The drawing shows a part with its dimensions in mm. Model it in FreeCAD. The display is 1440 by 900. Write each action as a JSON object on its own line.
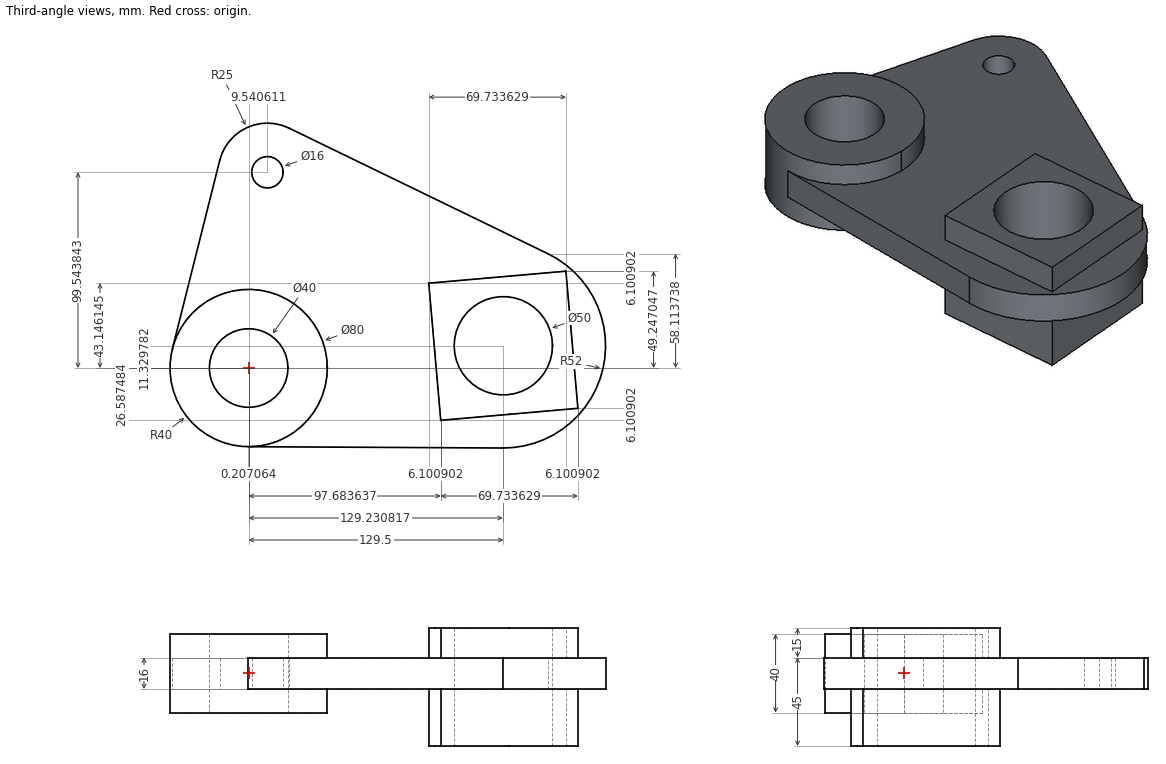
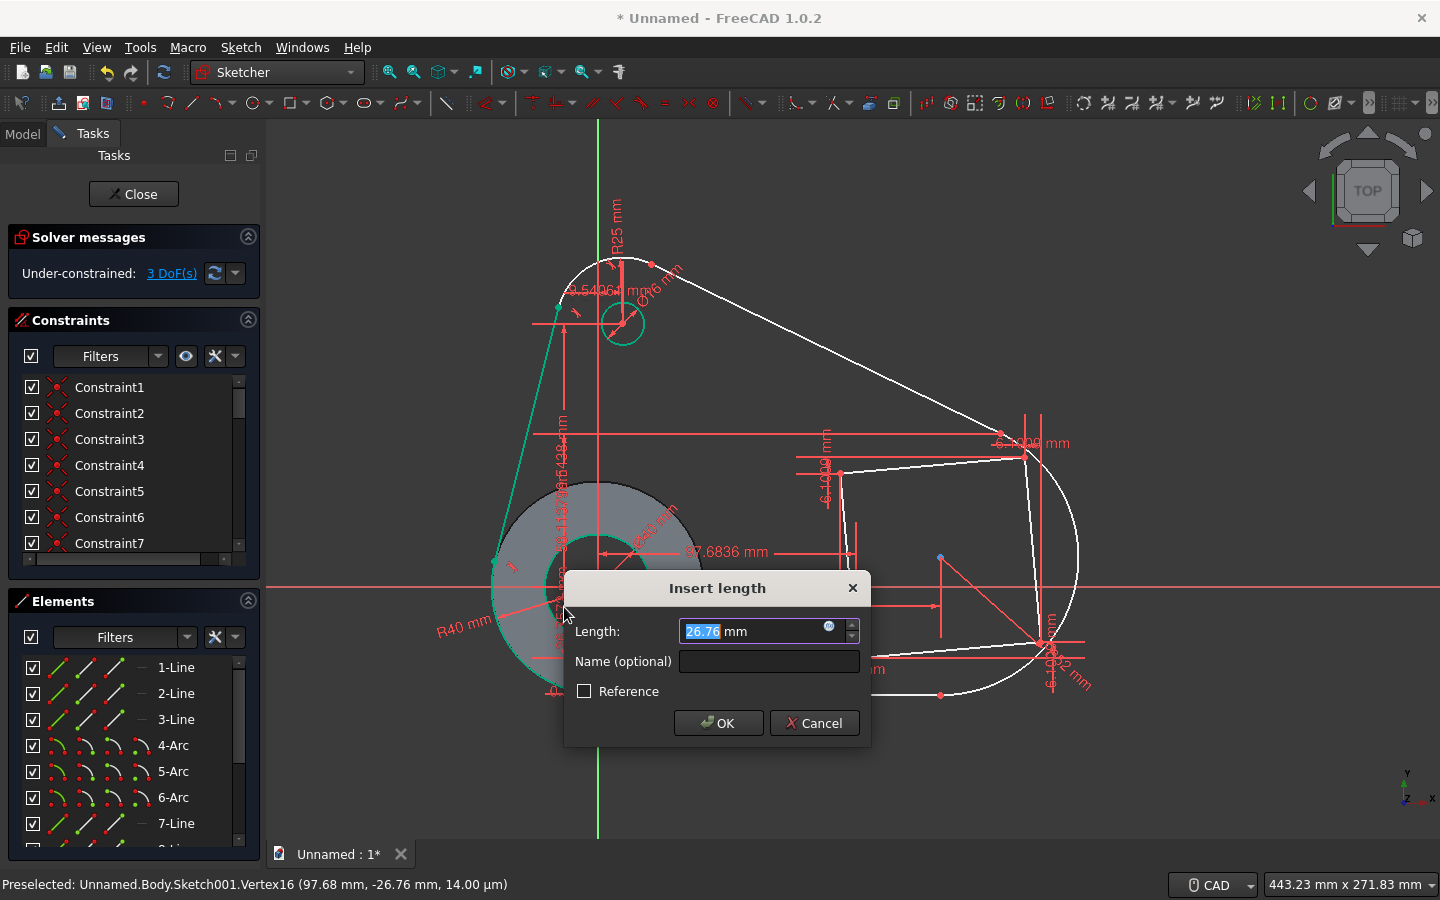
{"action": "type", "text": "26.587484"}
{"action": "key", "text": "Return"}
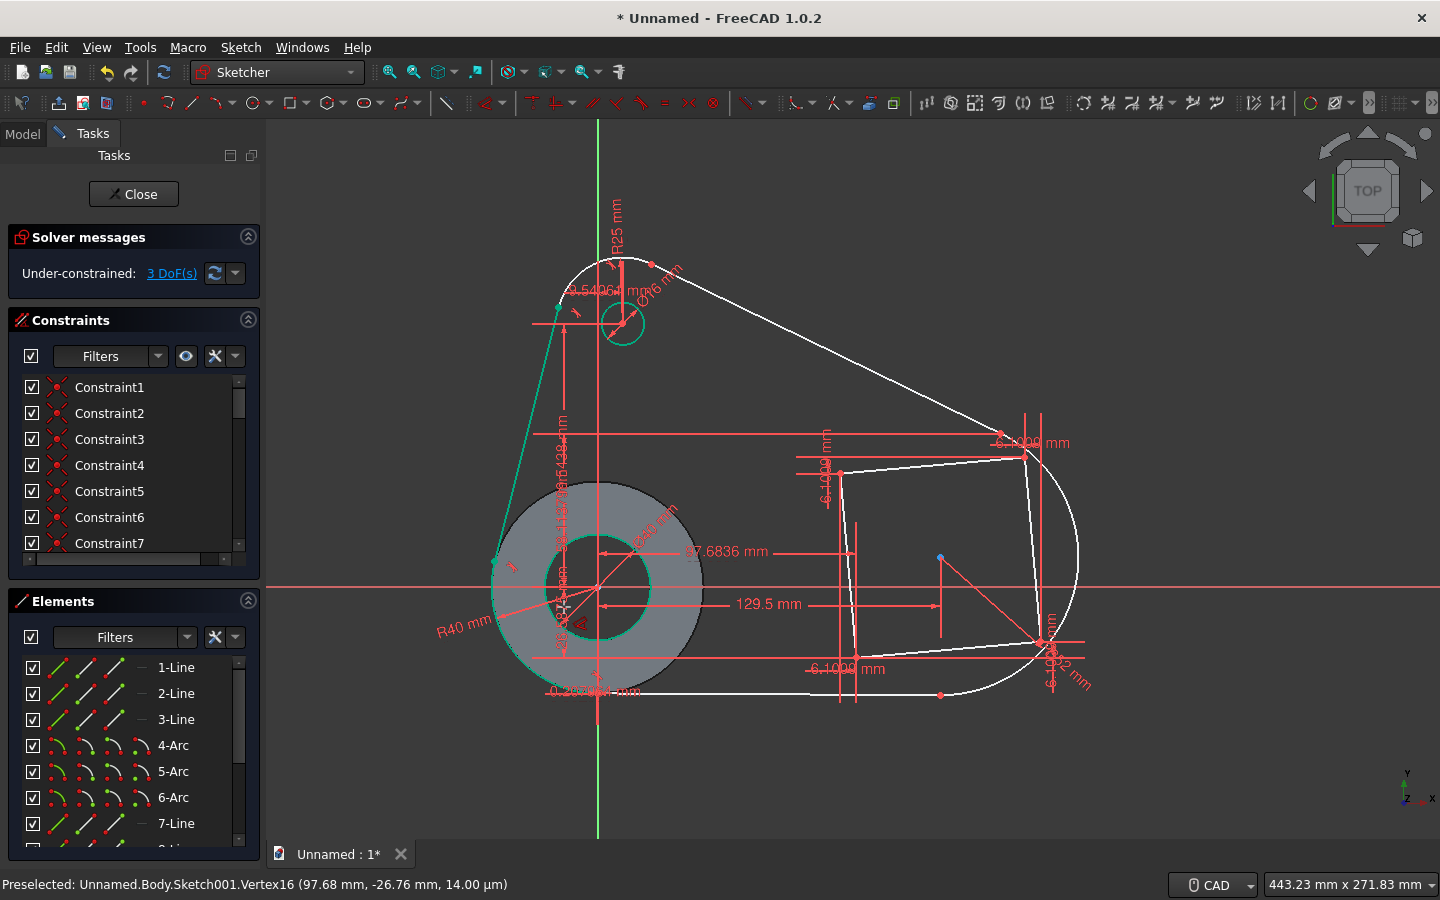
{"action": "left_click", "coordinate": [840, 474]}
{"action": "left_click", "coordinate": [564, 531]}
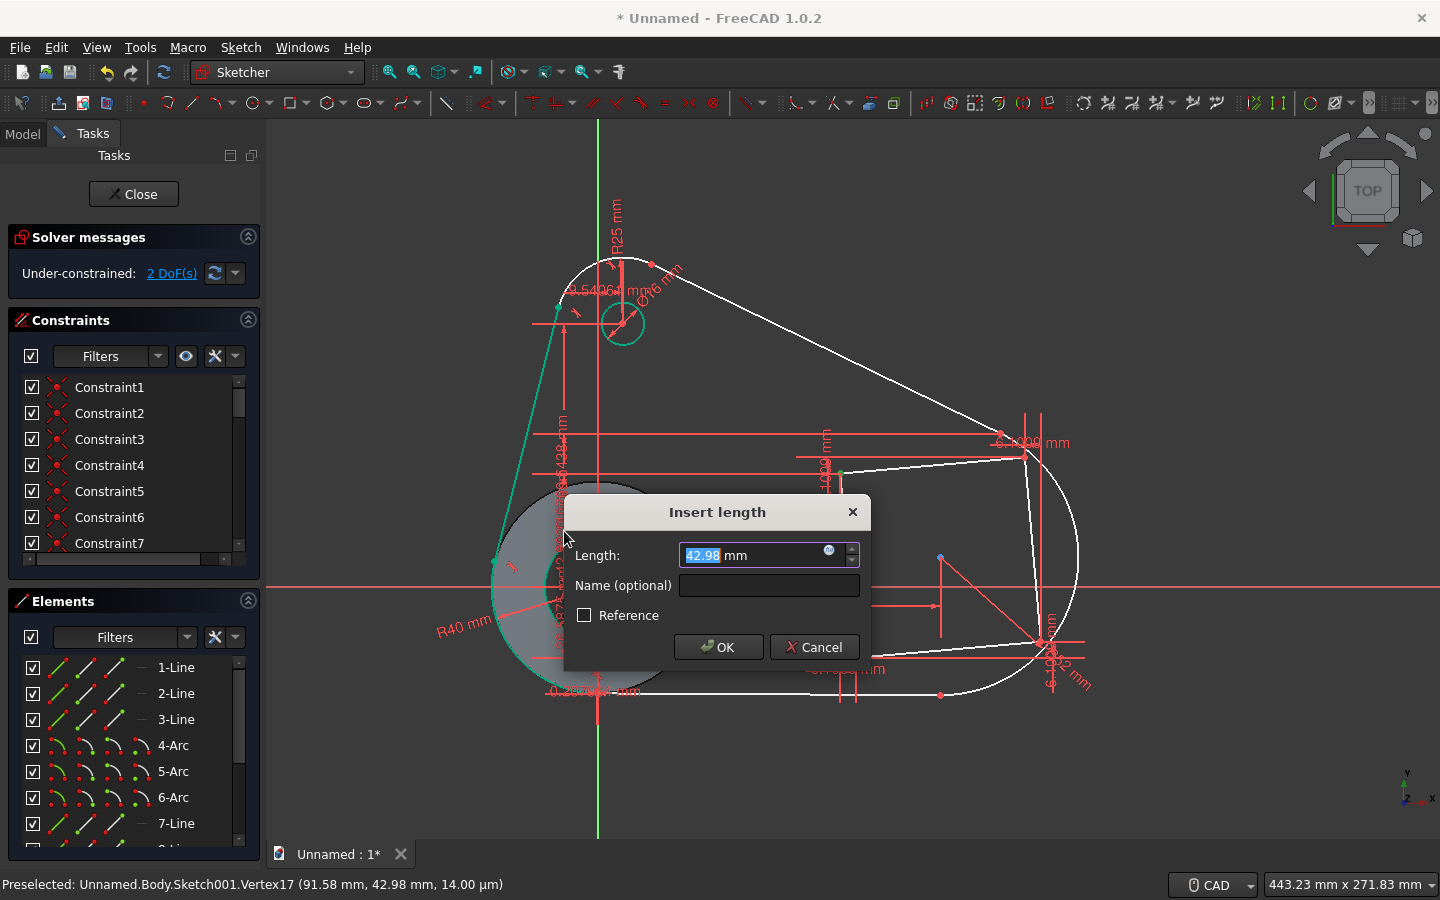
{"action": "type", "text": "43.146145"}
{"action": "key", "text": "Return"}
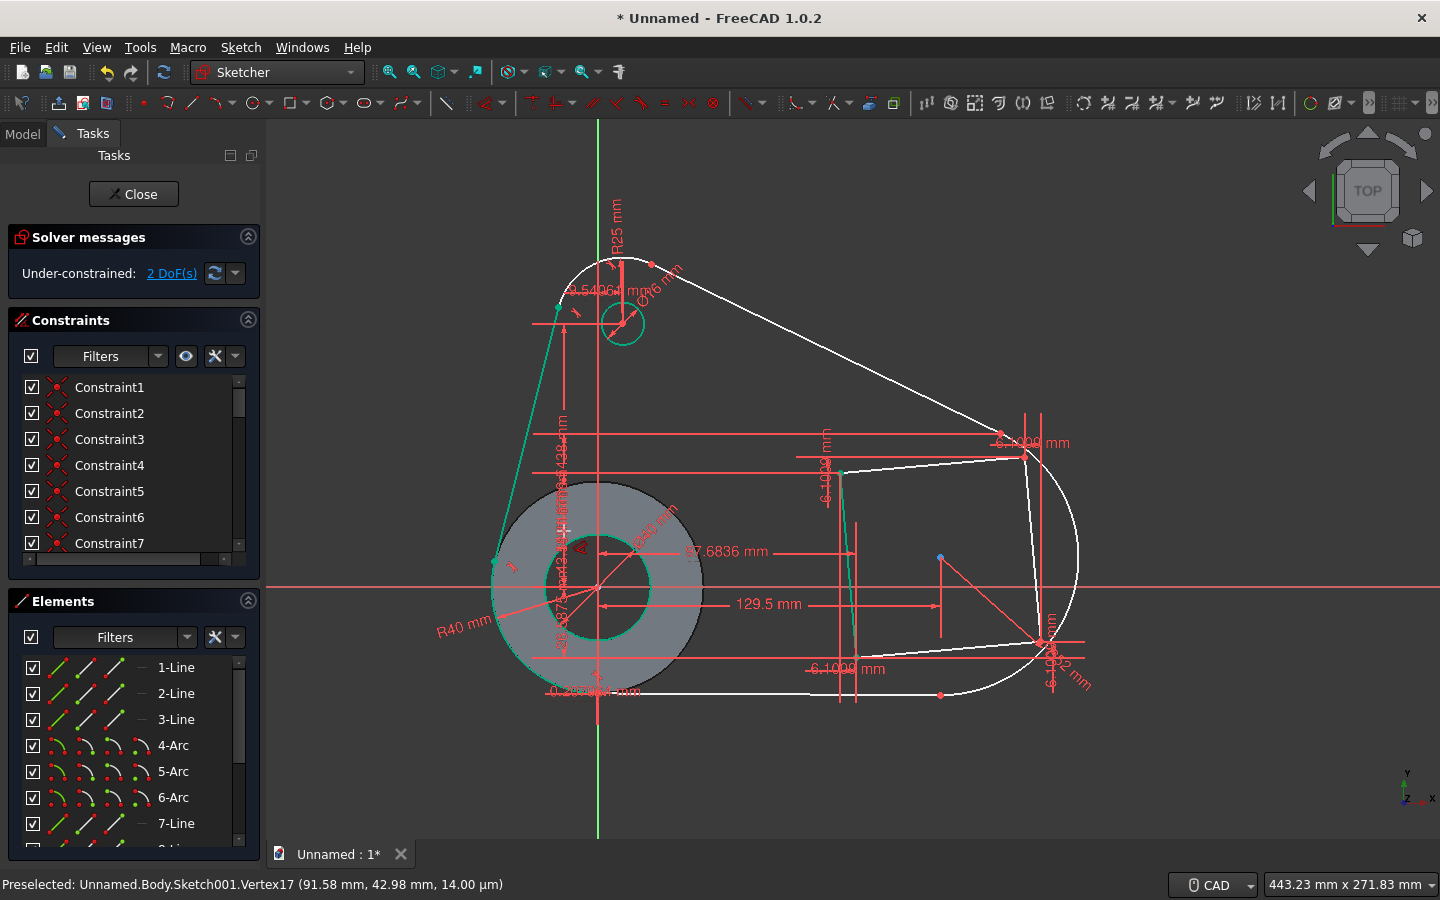
{"action": "left_click", "coordinate": [896, 468]}
{"action": "left_click", "coordinate": [933, 423]}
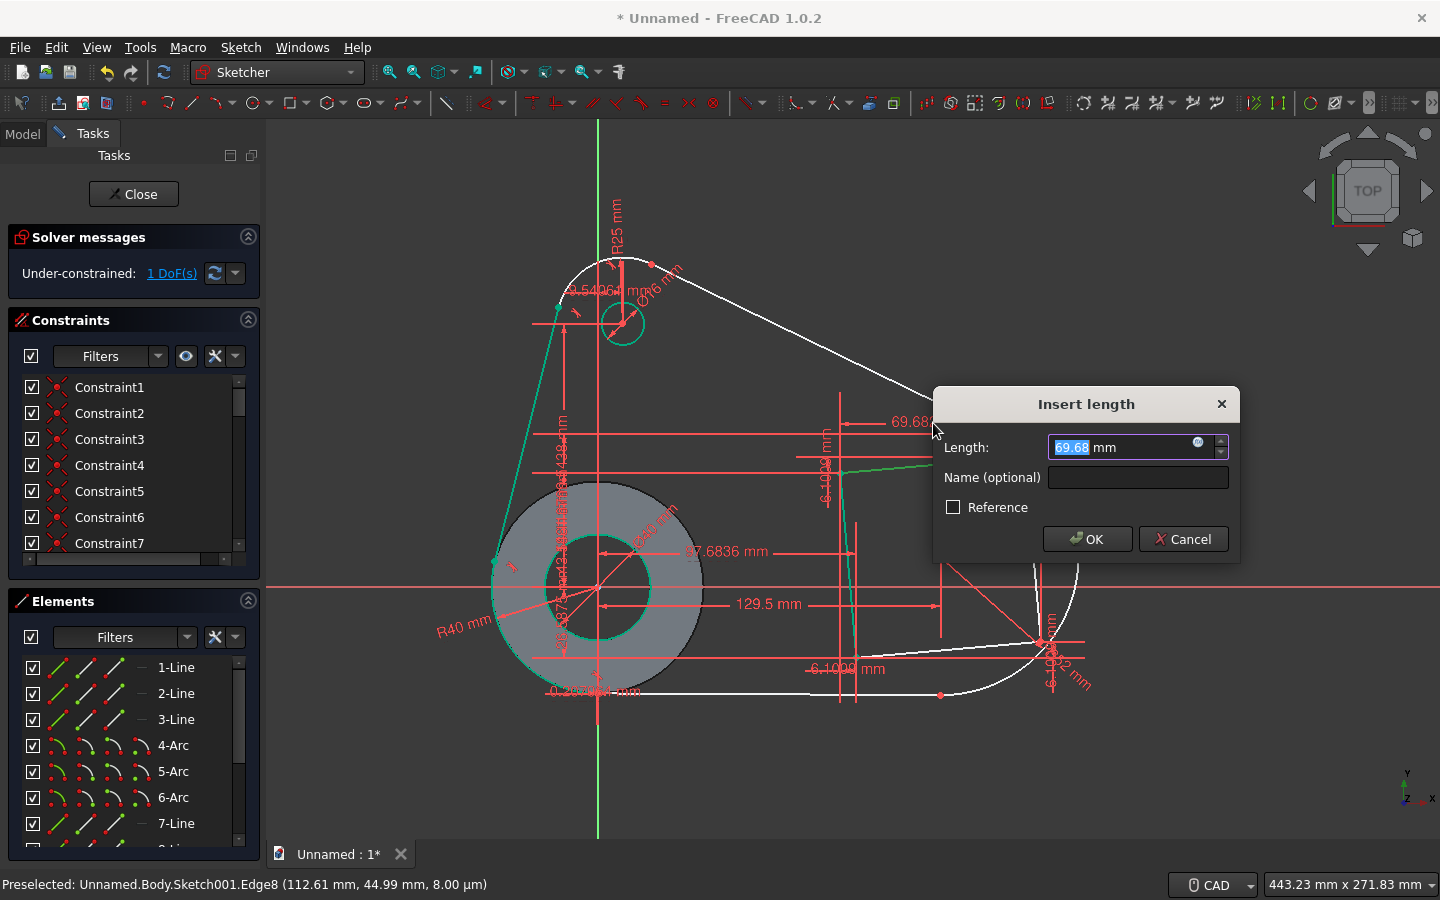
{"action": "type", "text": "69.733629"}
{"action": "key", "text": "Return"}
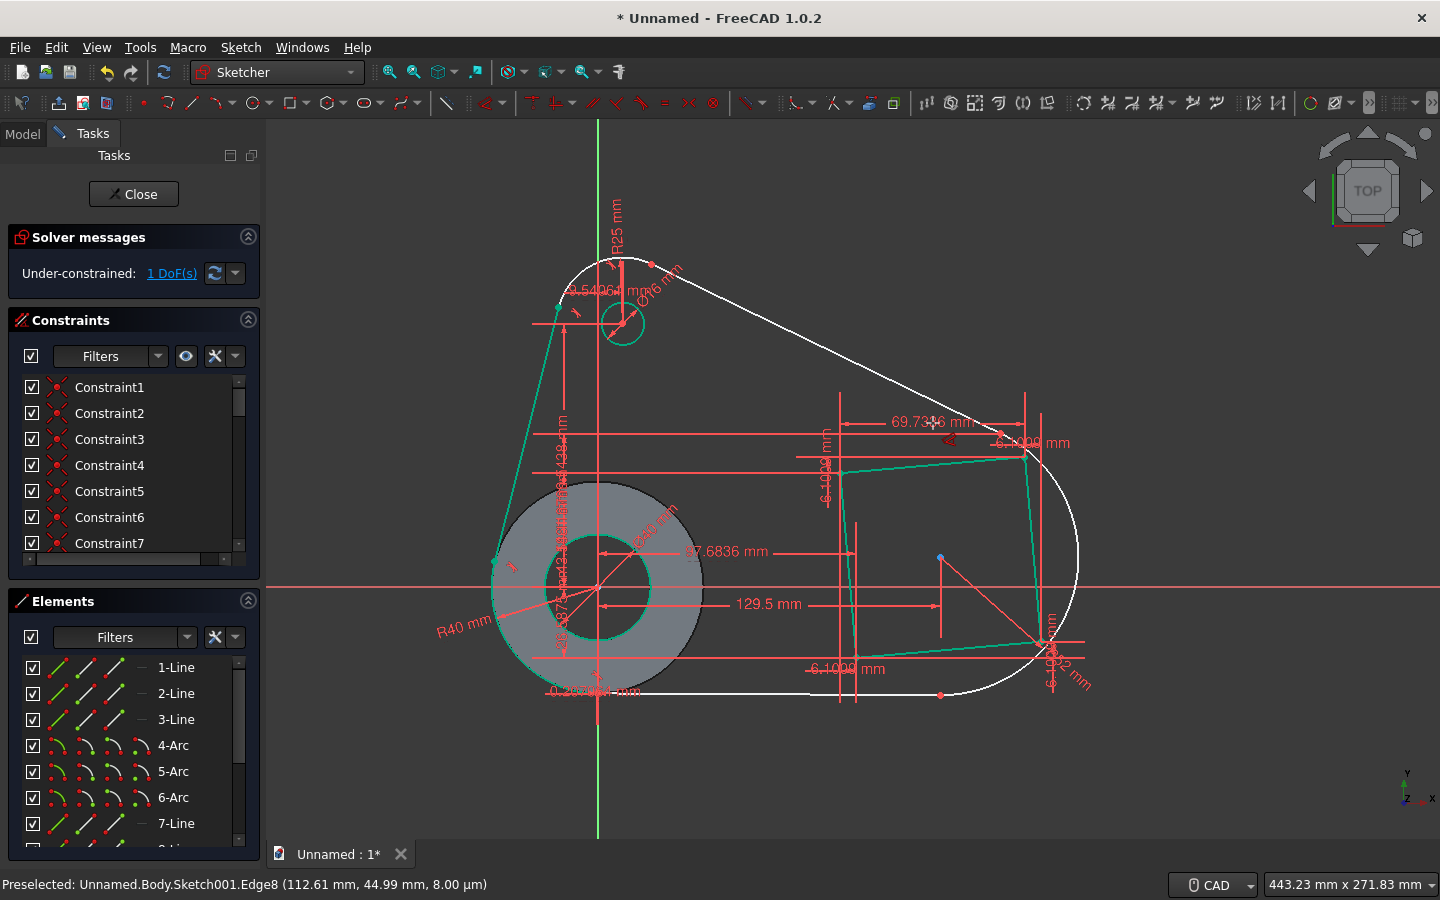
{"action": "left_click", "coordinate": [940, 695]}
{"action": "left_click", "coordinate": [769, 729]}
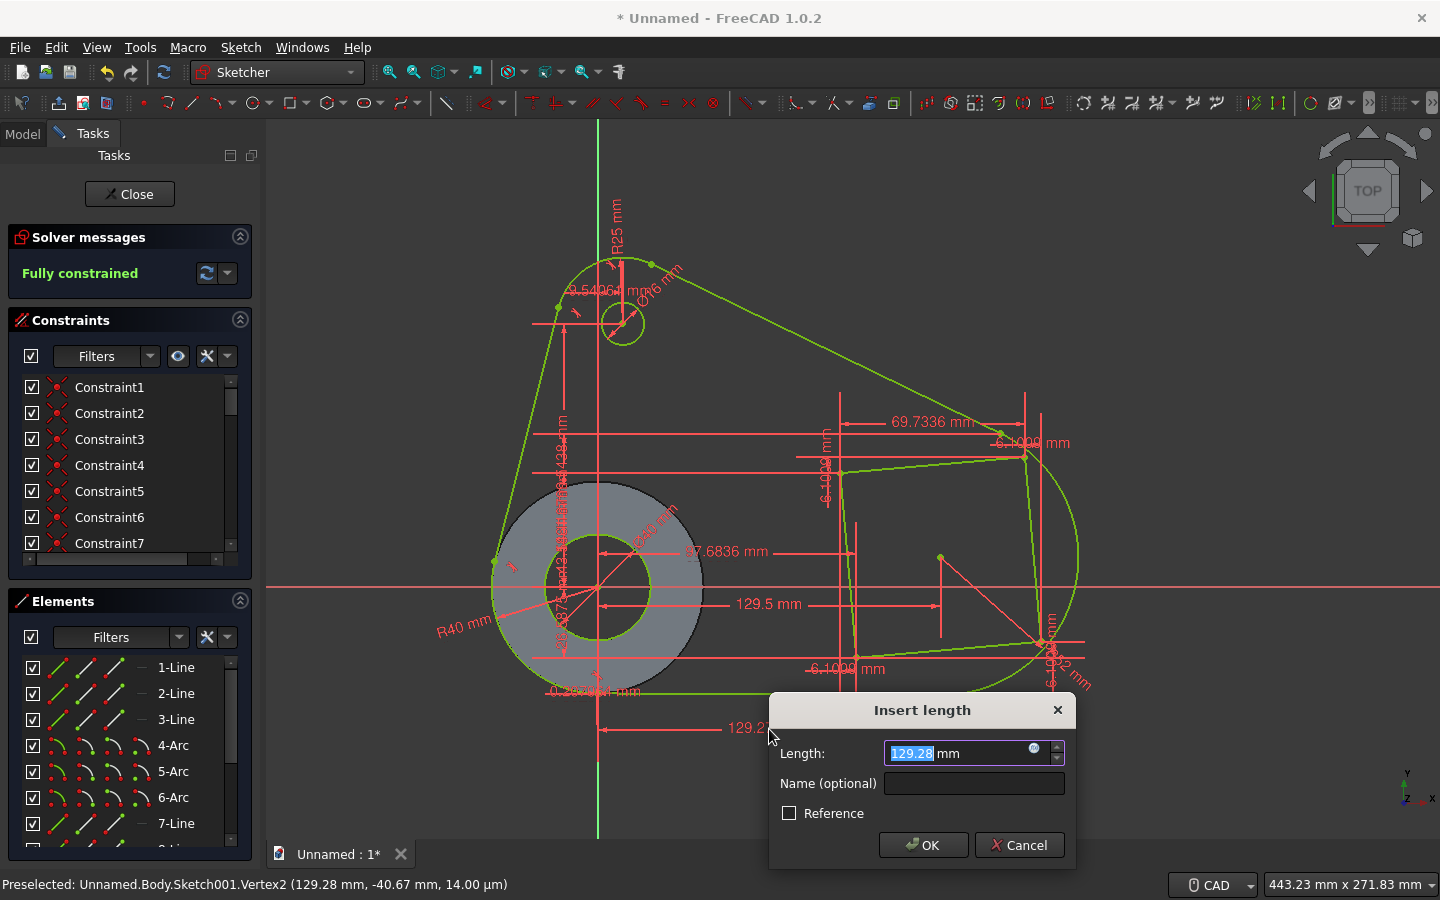
{"action": "type", "text": "129.230817"}
{"action": "key", "text": "Return"}
{"action": "key", "text": "Escape"}